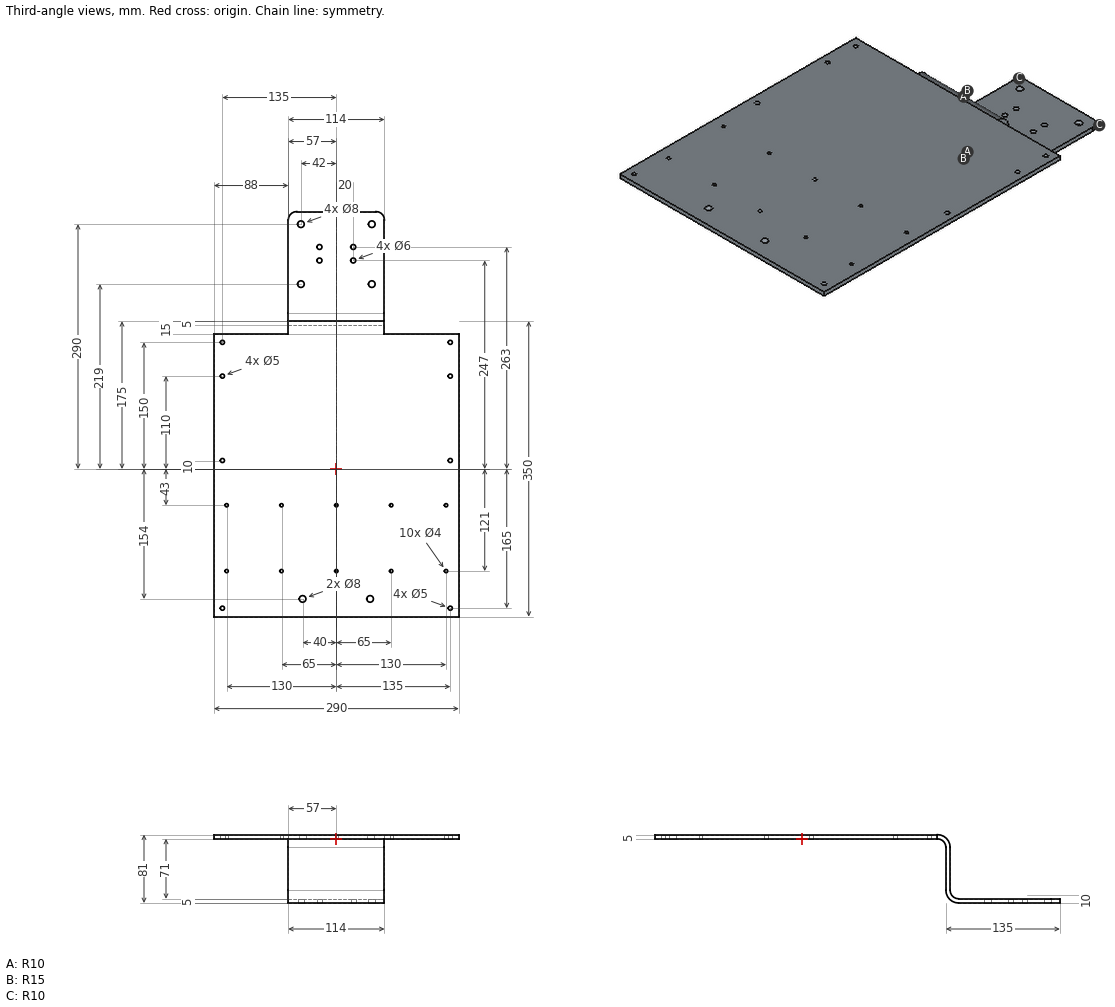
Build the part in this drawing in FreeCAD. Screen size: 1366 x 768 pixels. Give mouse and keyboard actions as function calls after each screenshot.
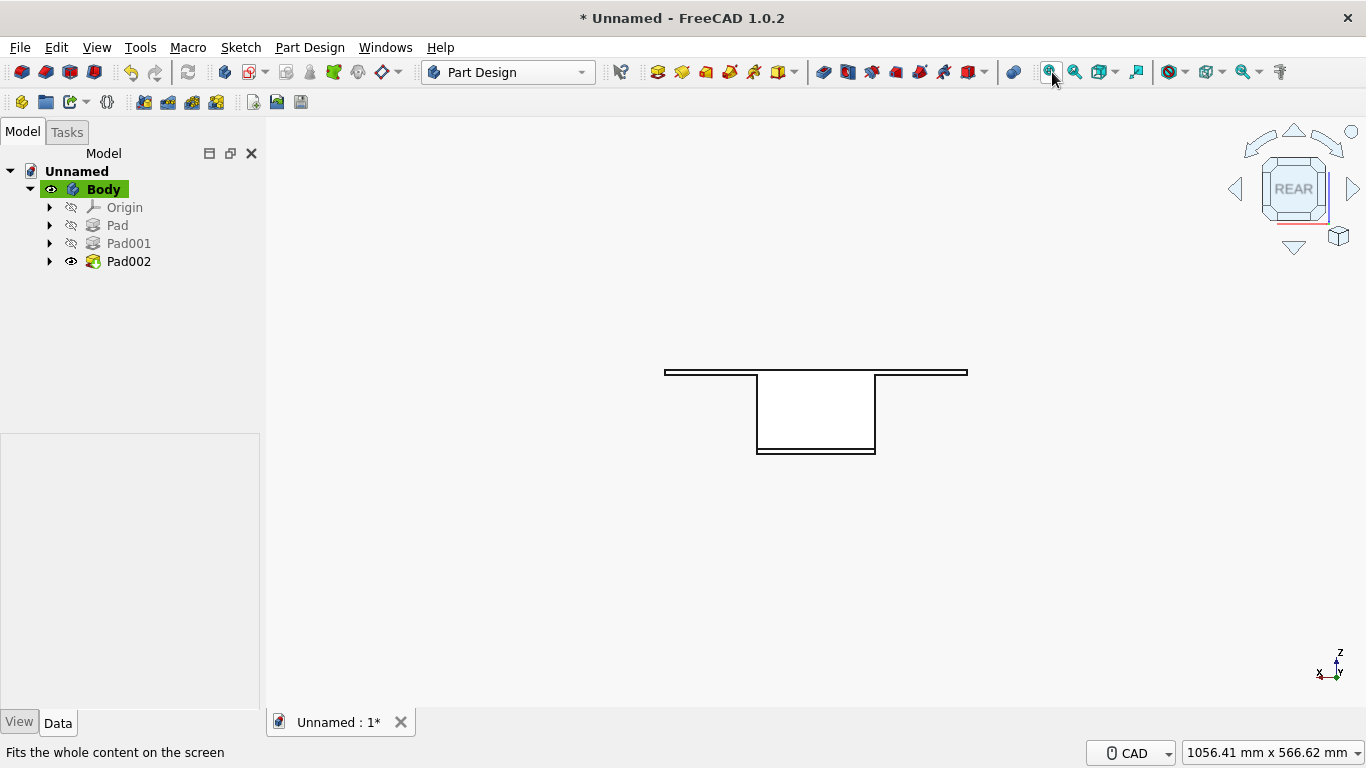
key(6)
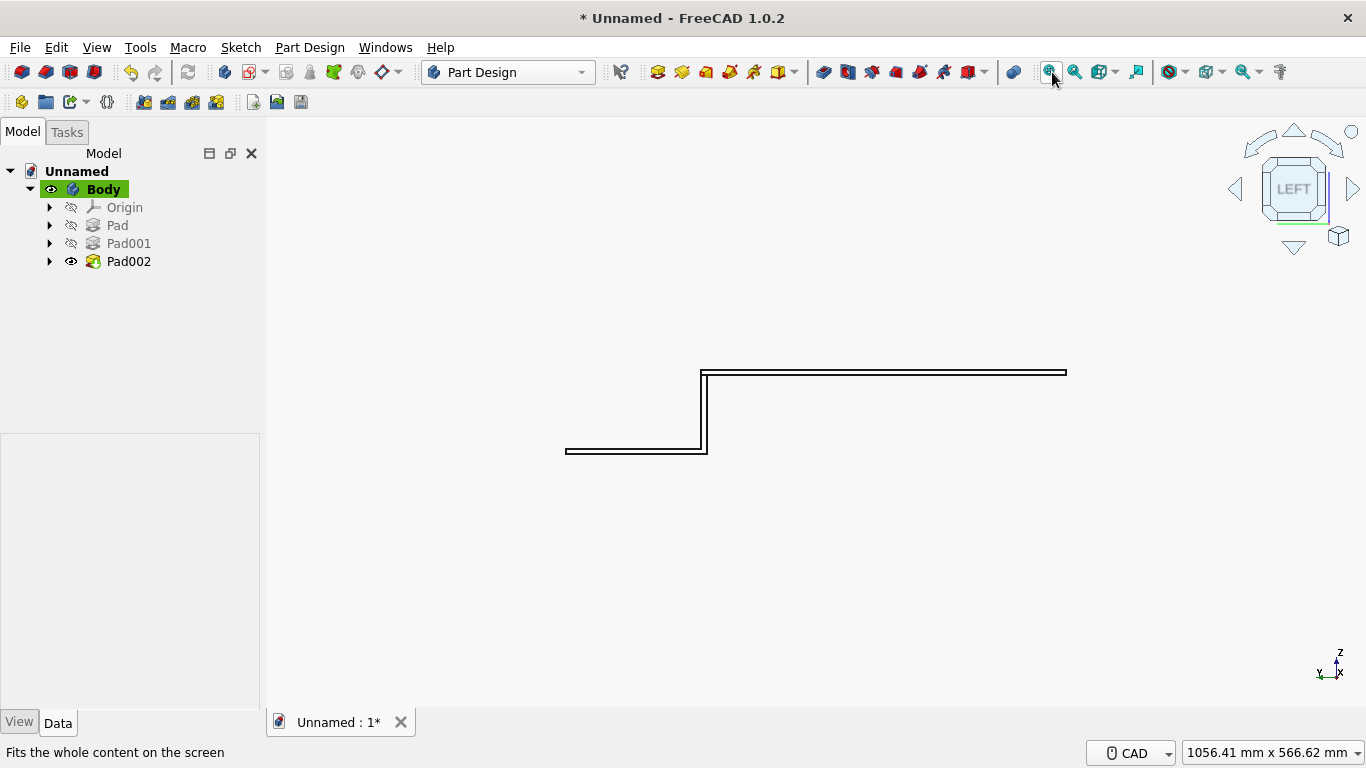
key(v)
key(3)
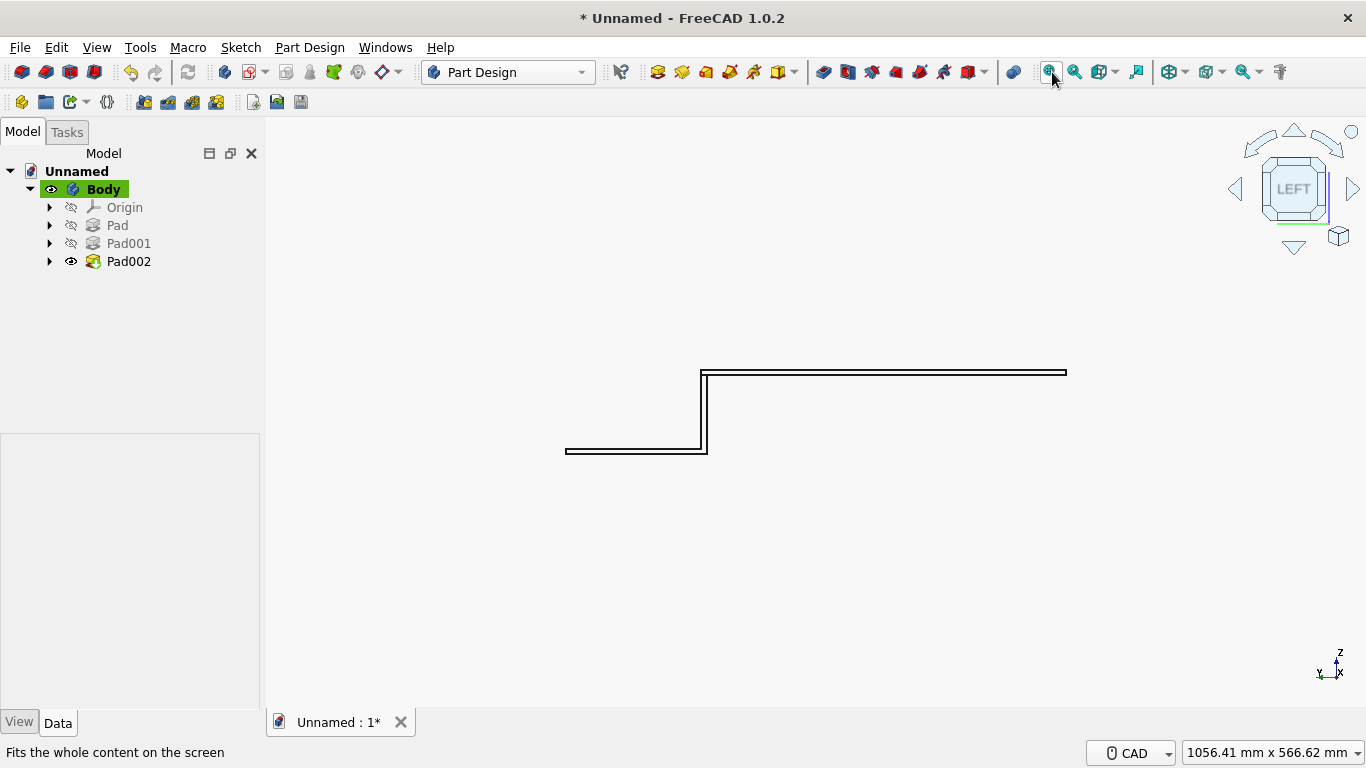
key(0)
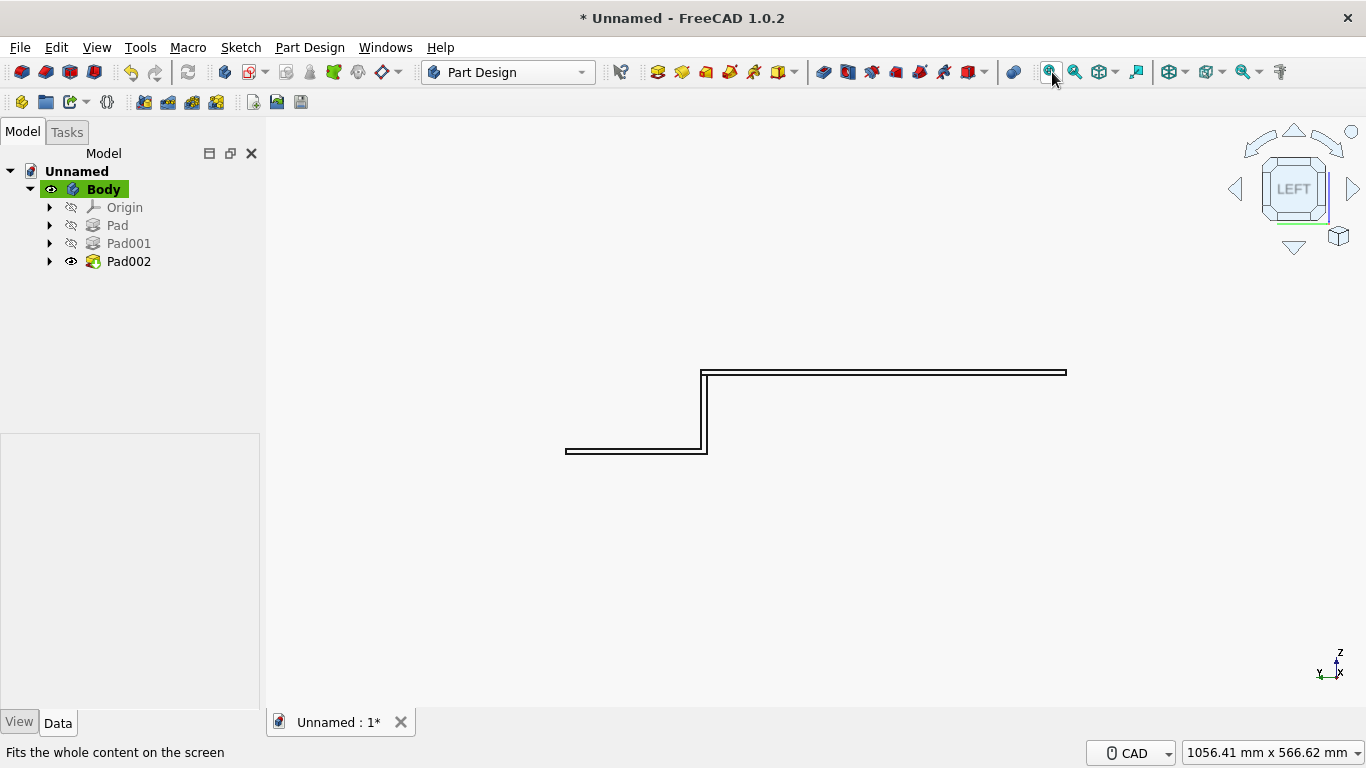
click(893, 336)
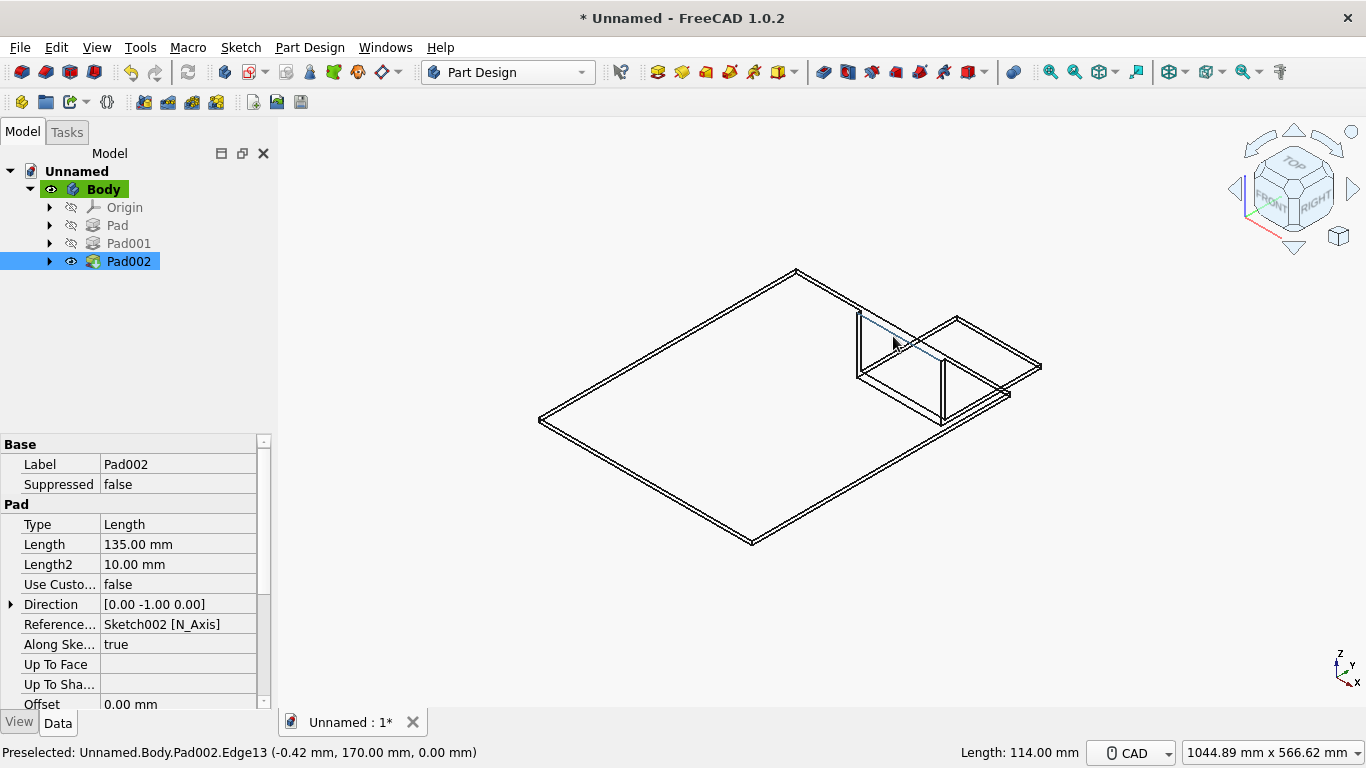
click(903, 394, ctrl)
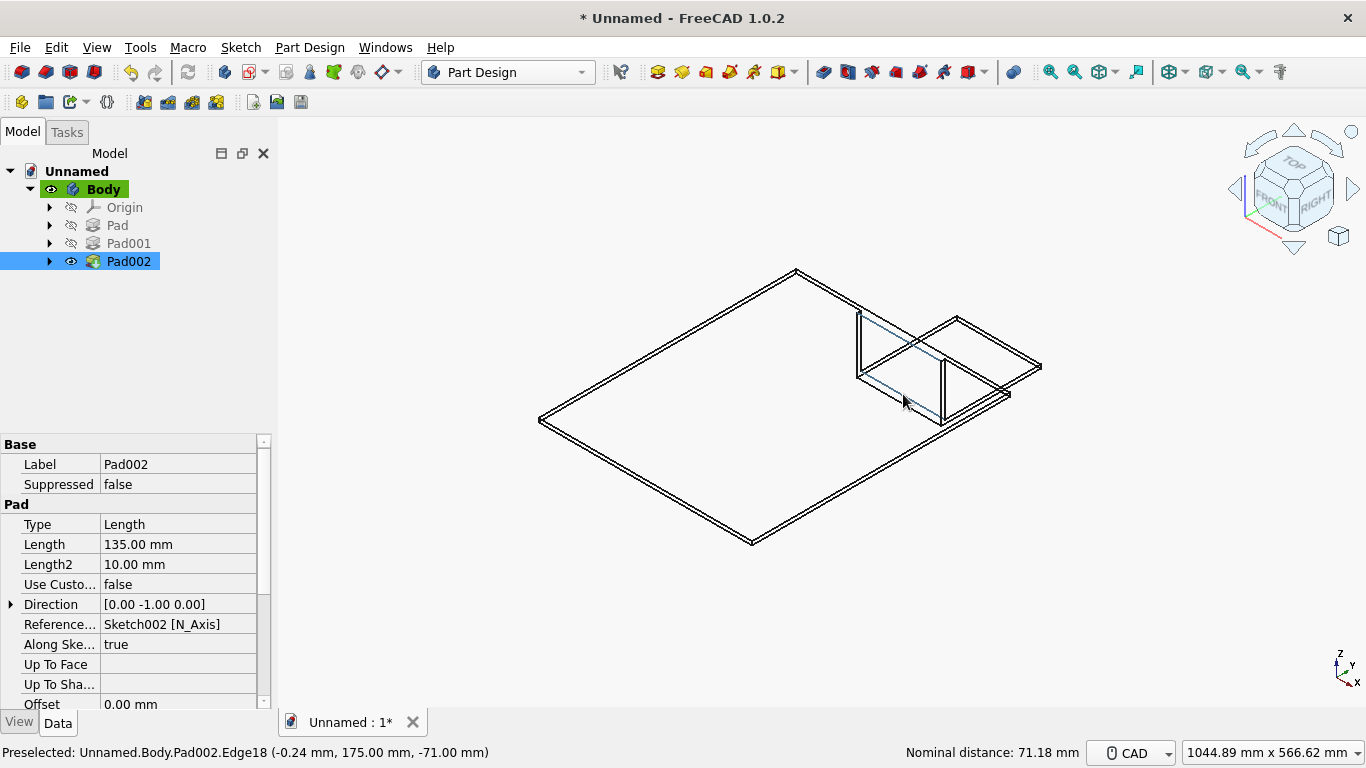
key(v)
key(1)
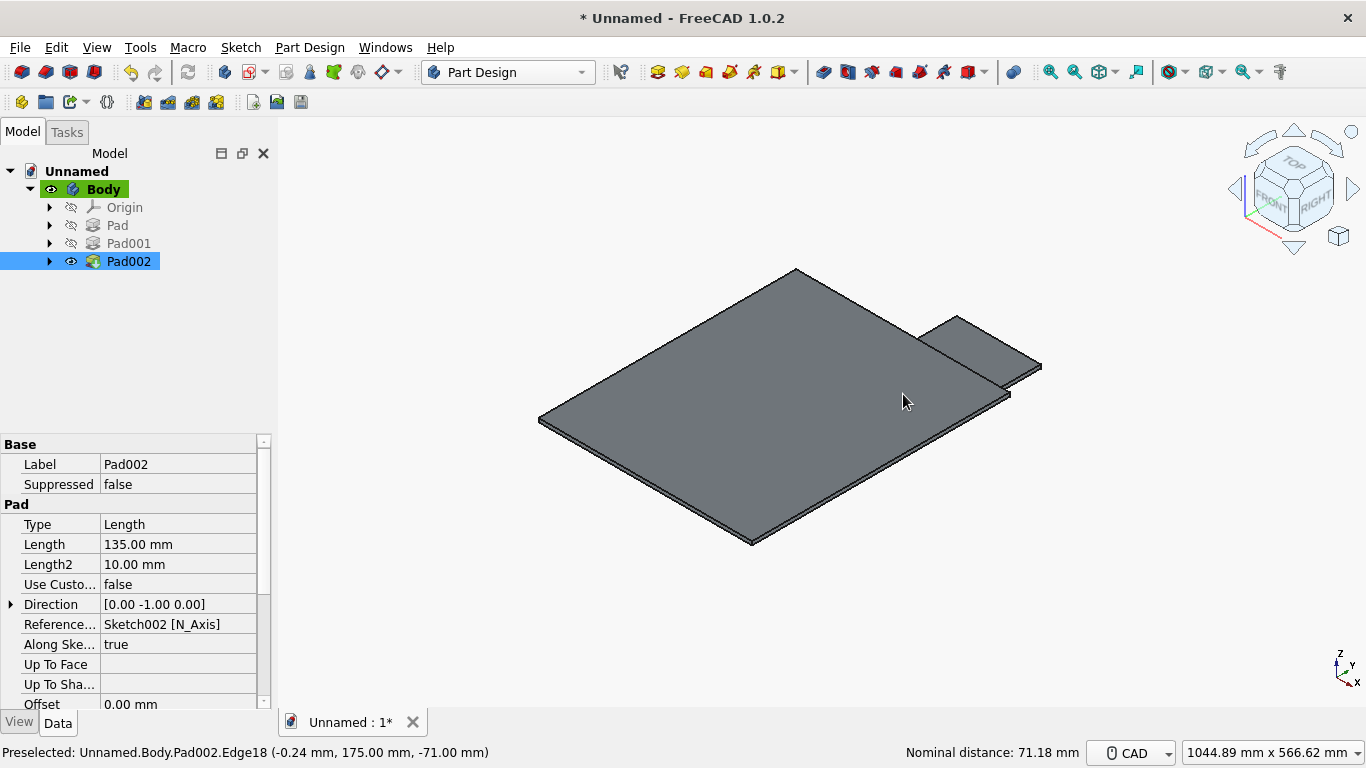
click(22, 72)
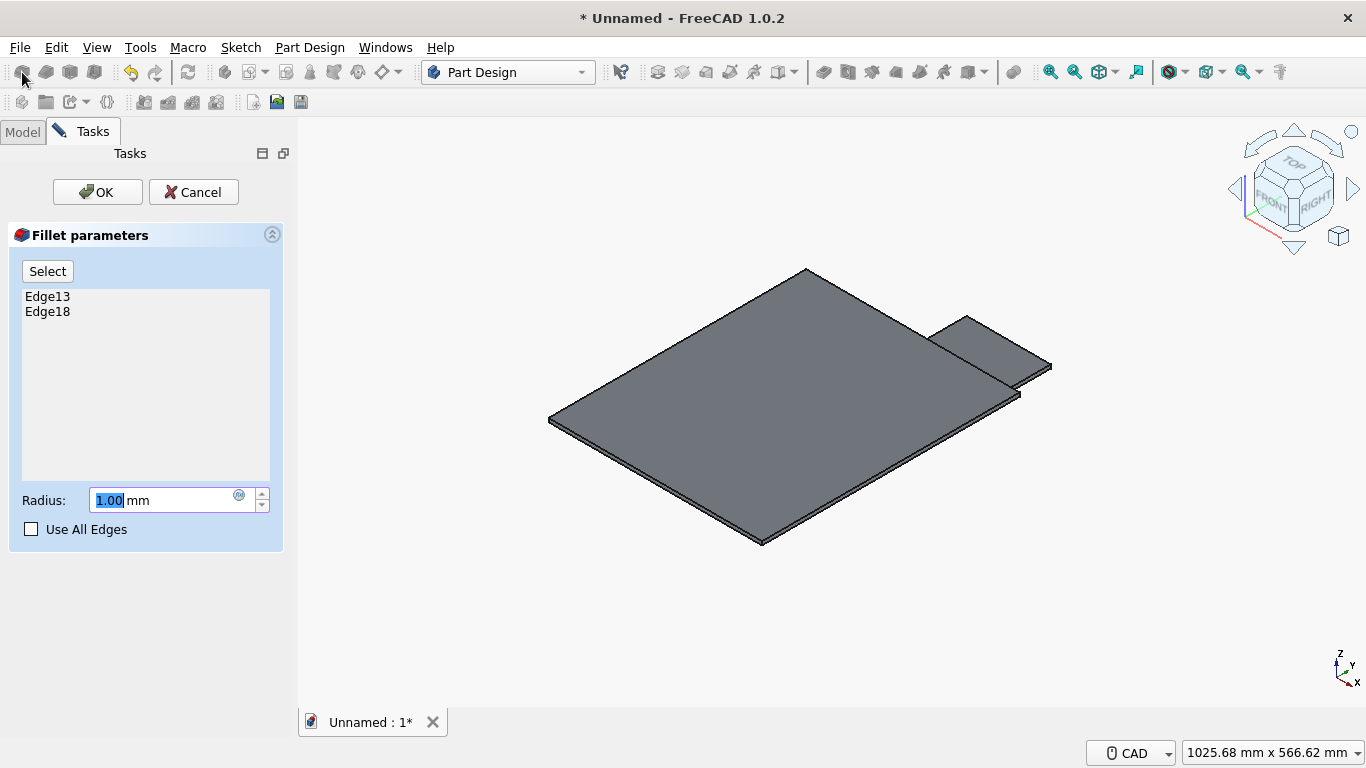
text(10)
key(Tab)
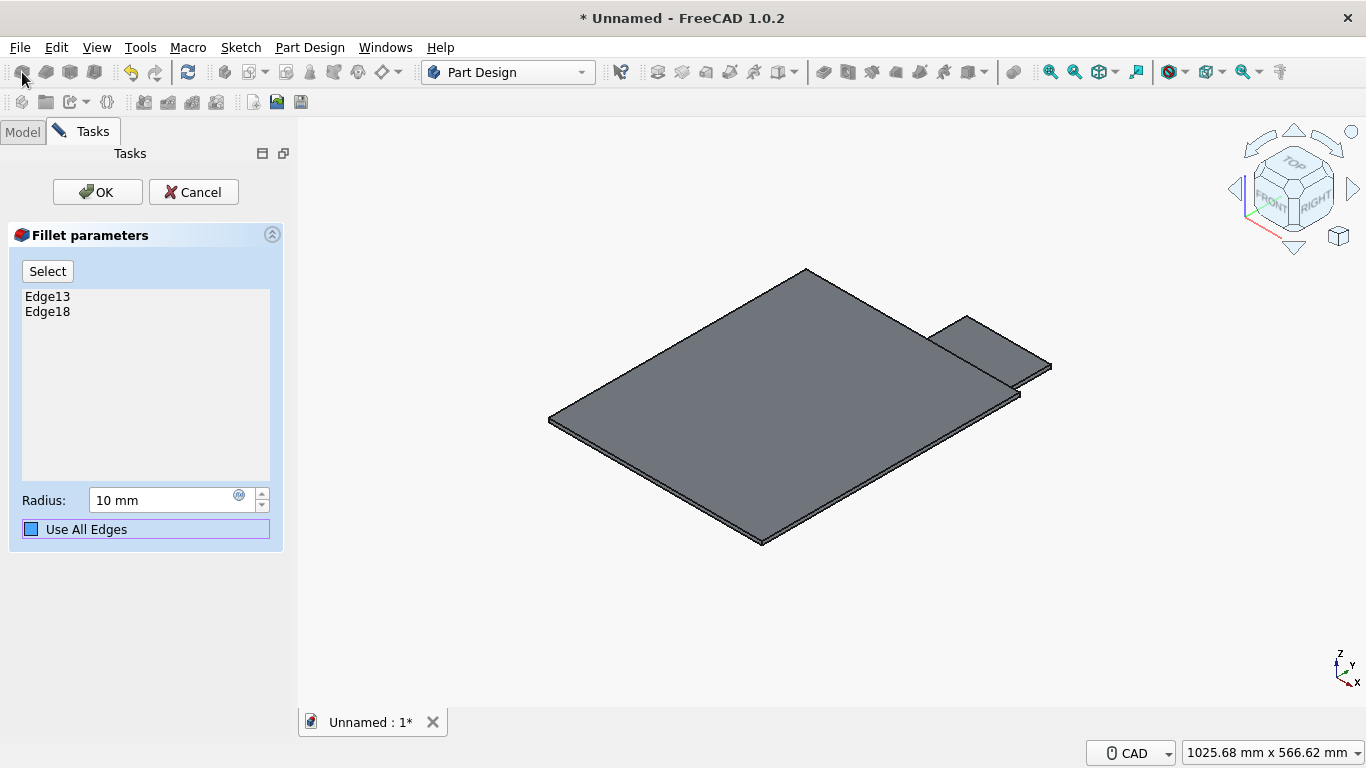
click(98, 192)